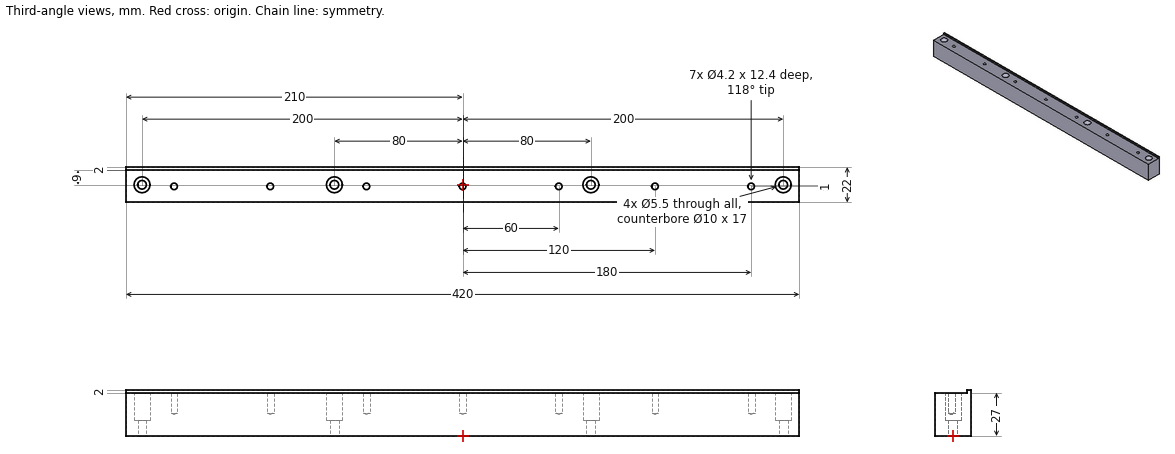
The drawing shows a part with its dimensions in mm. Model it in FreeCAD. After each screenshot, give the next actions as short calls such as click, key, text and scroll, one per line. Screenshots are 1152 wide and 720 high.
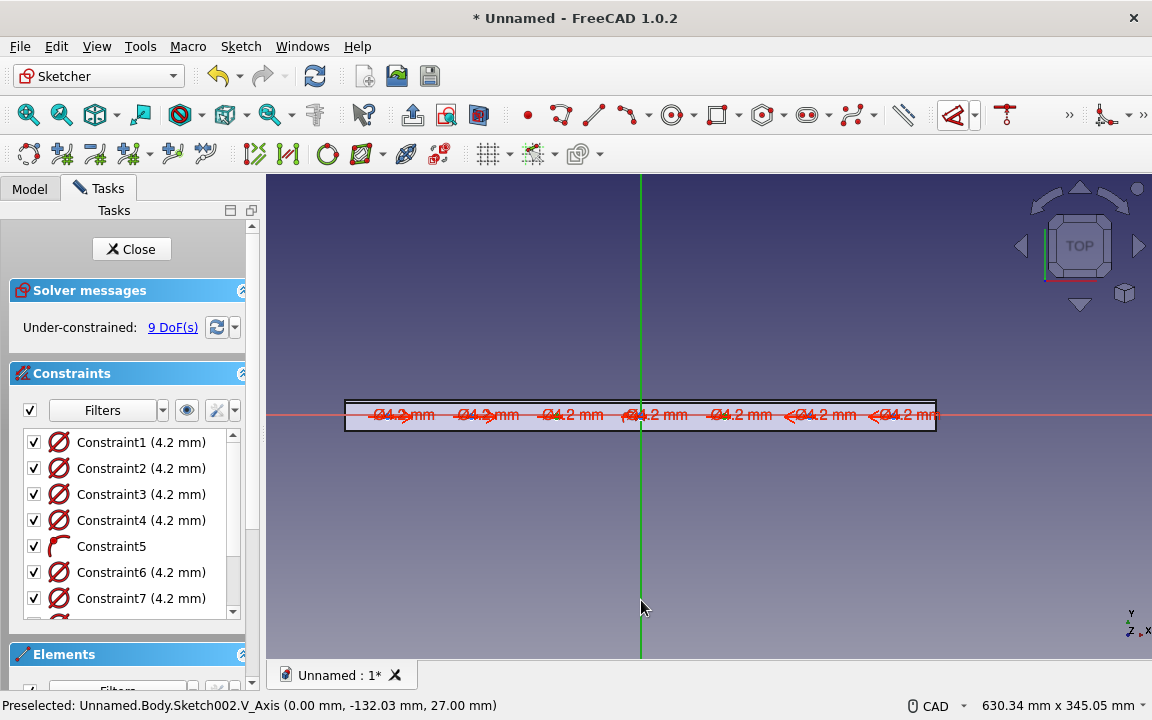
key(s)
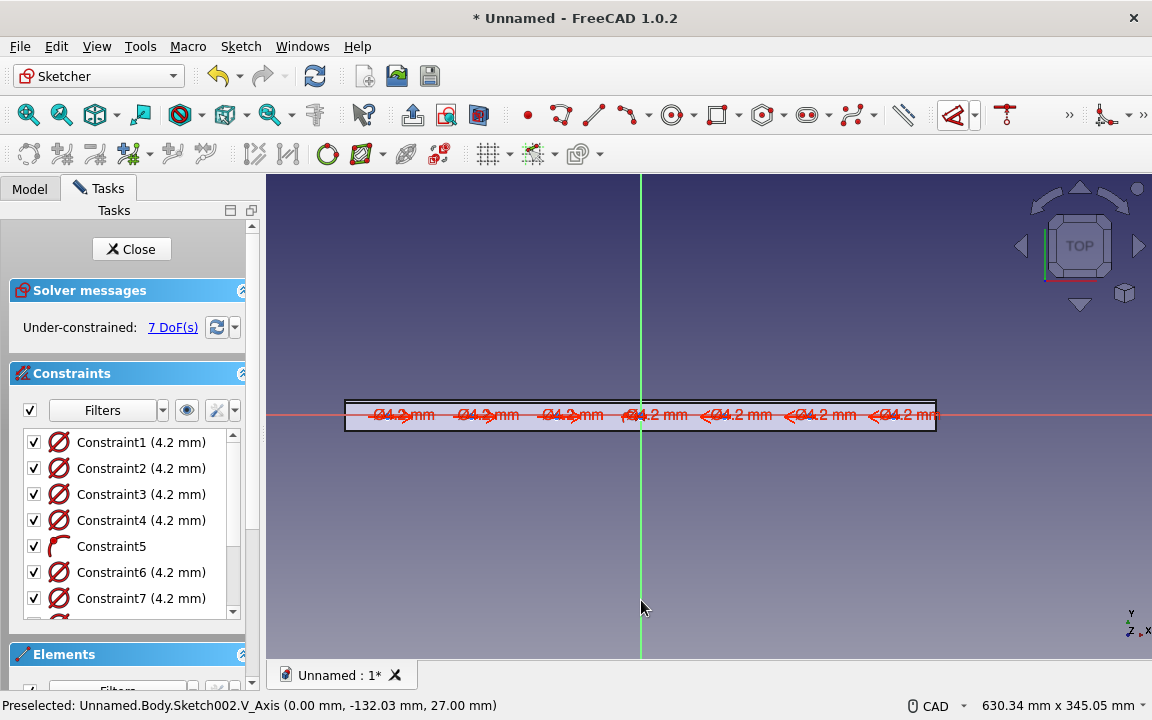
key(d)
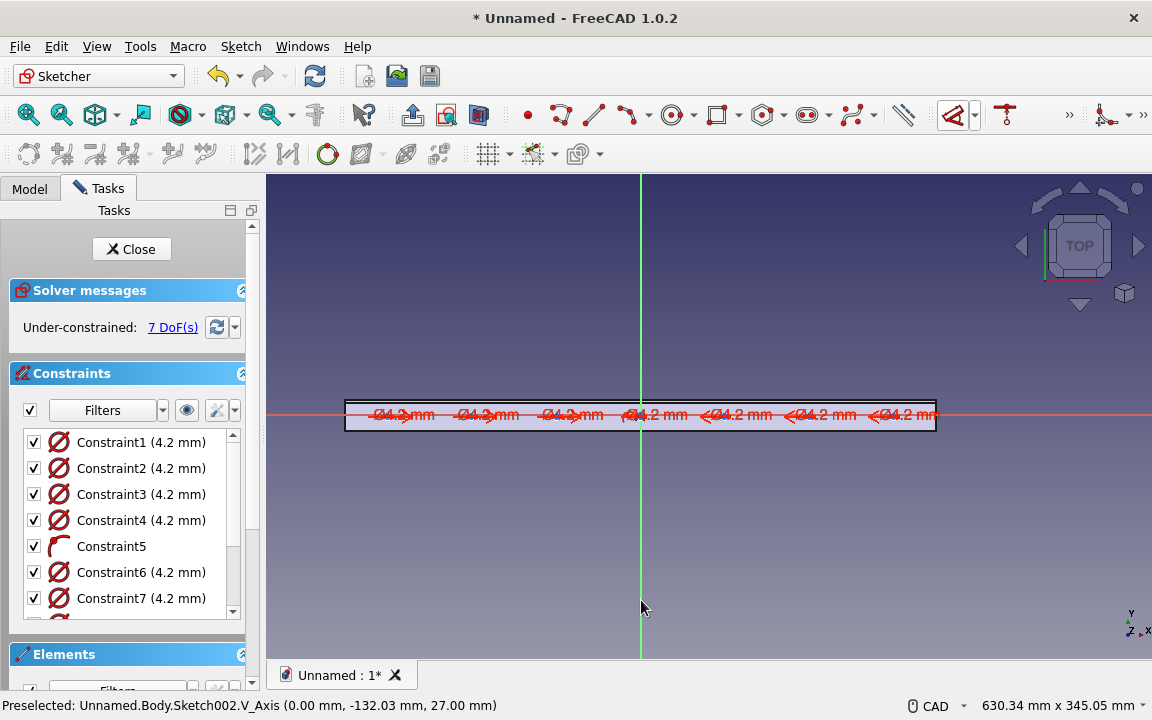
scroll(894, 417, up, 17)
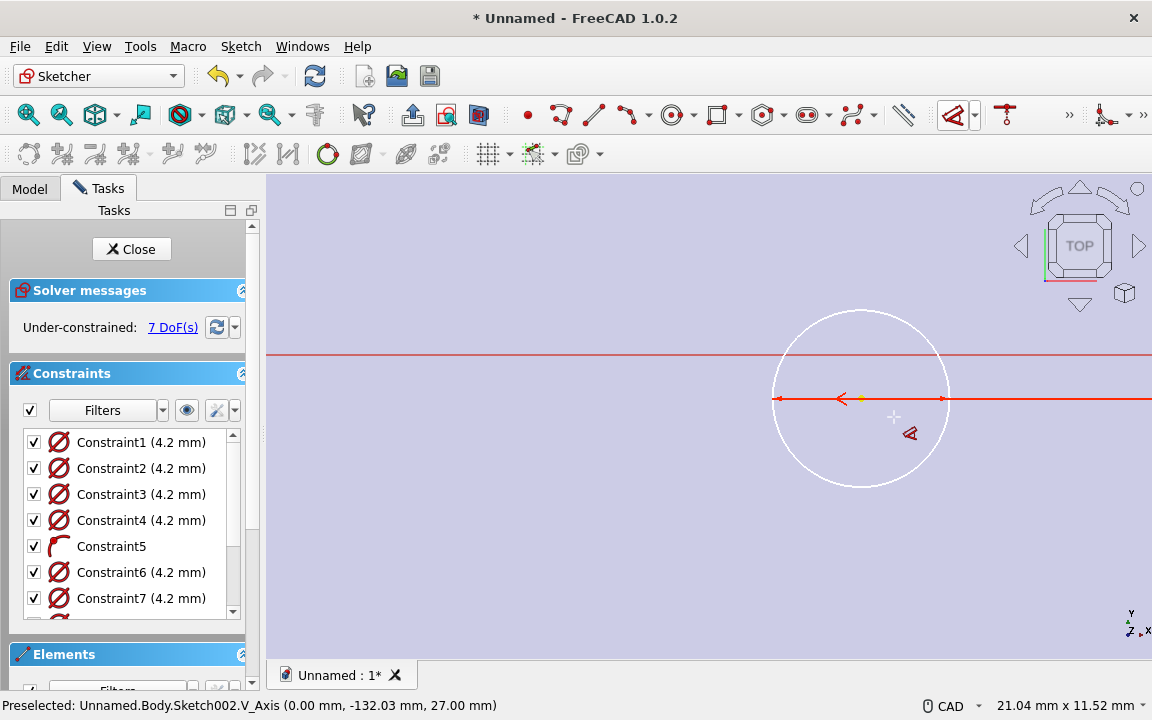
click(861, 399)
click(895, 377)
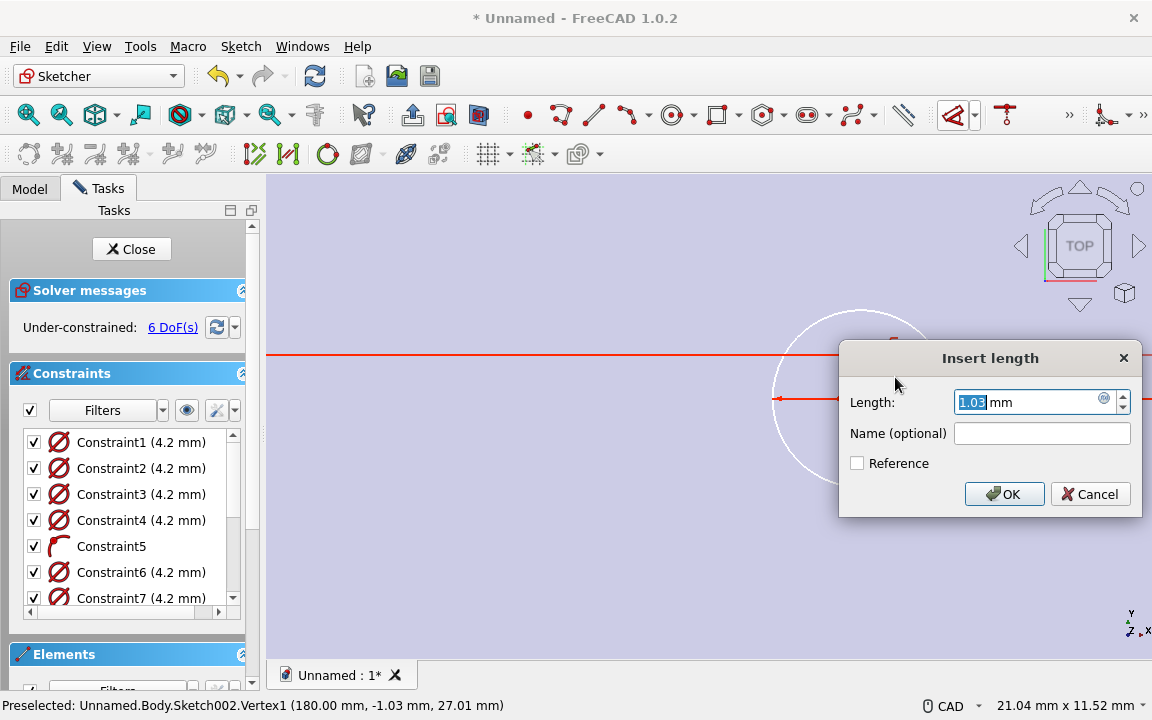
text(1)
key(Return)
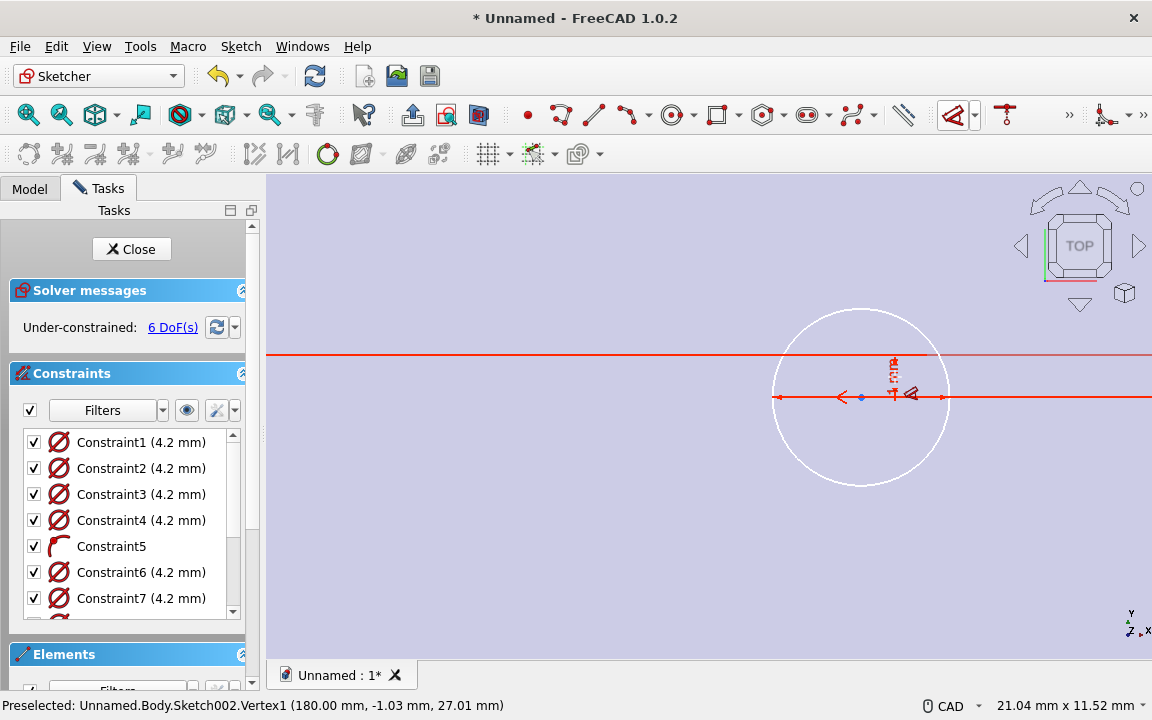
scroll(953, 417, down, 16)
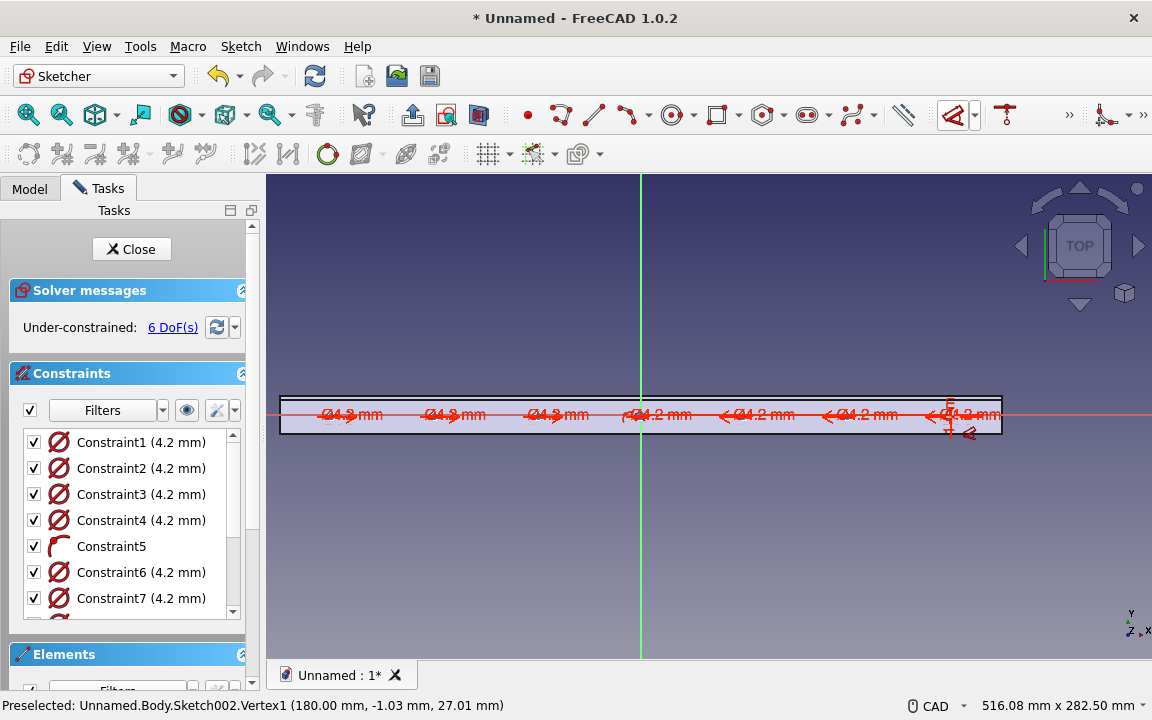
scroll(847, 417, up, 16)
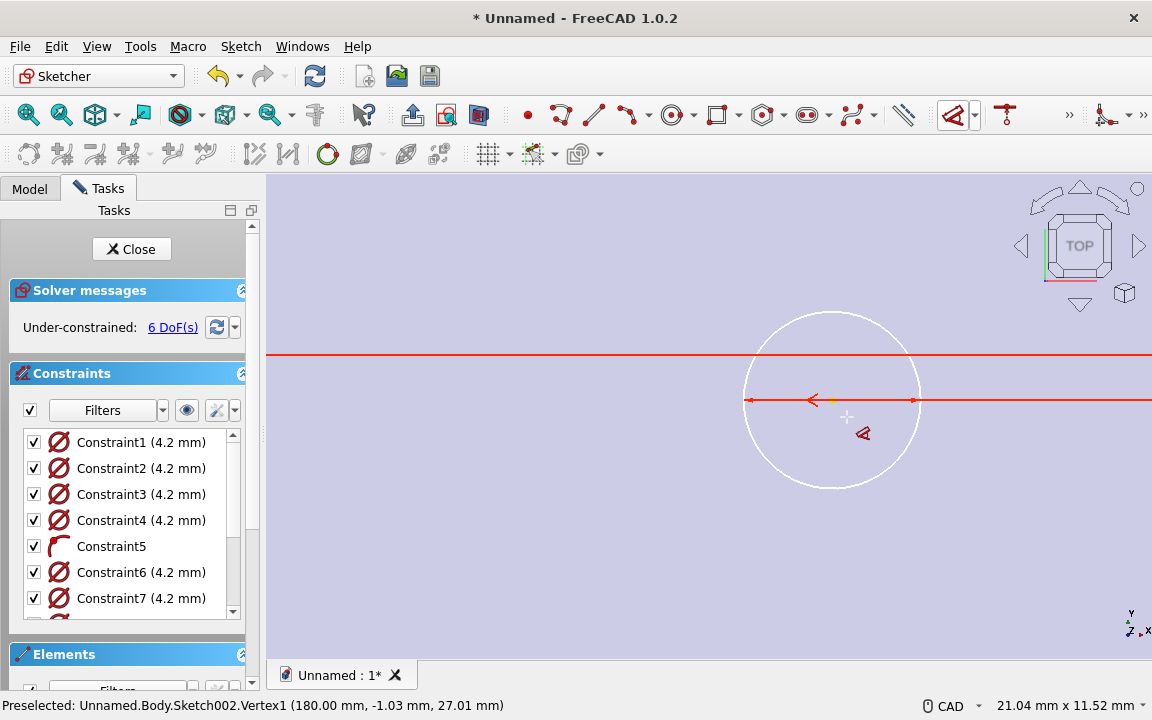
click(832, 400)
click(866, 378)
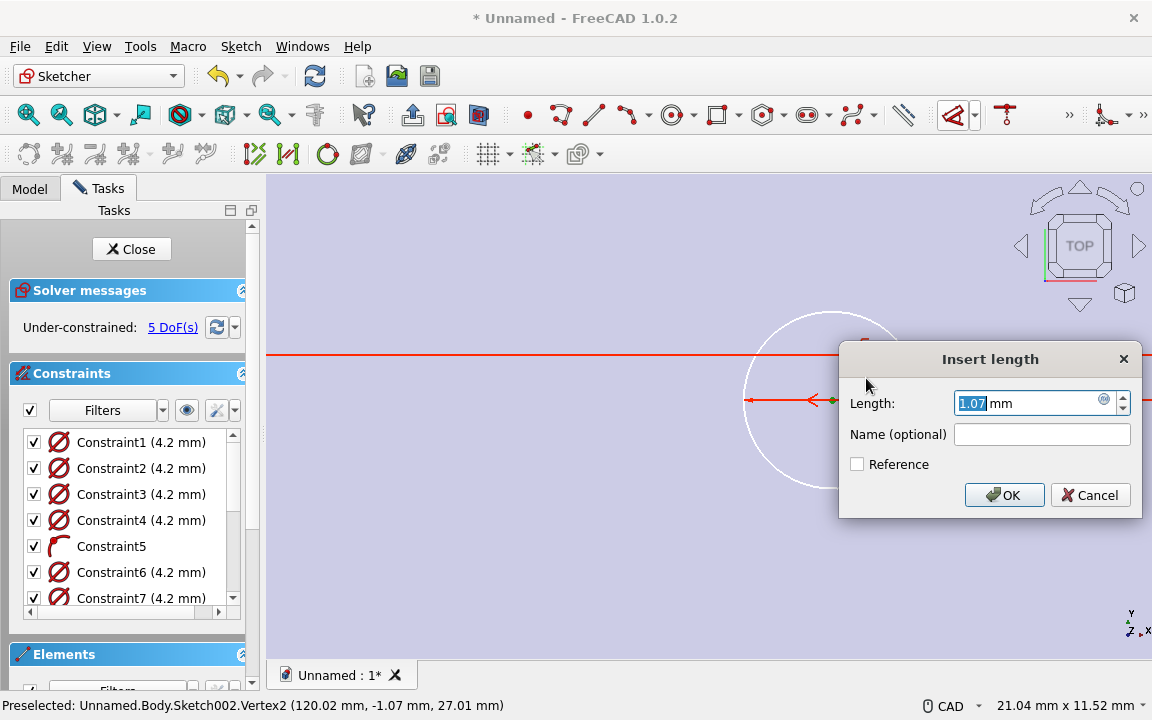
text(1)
key(Return)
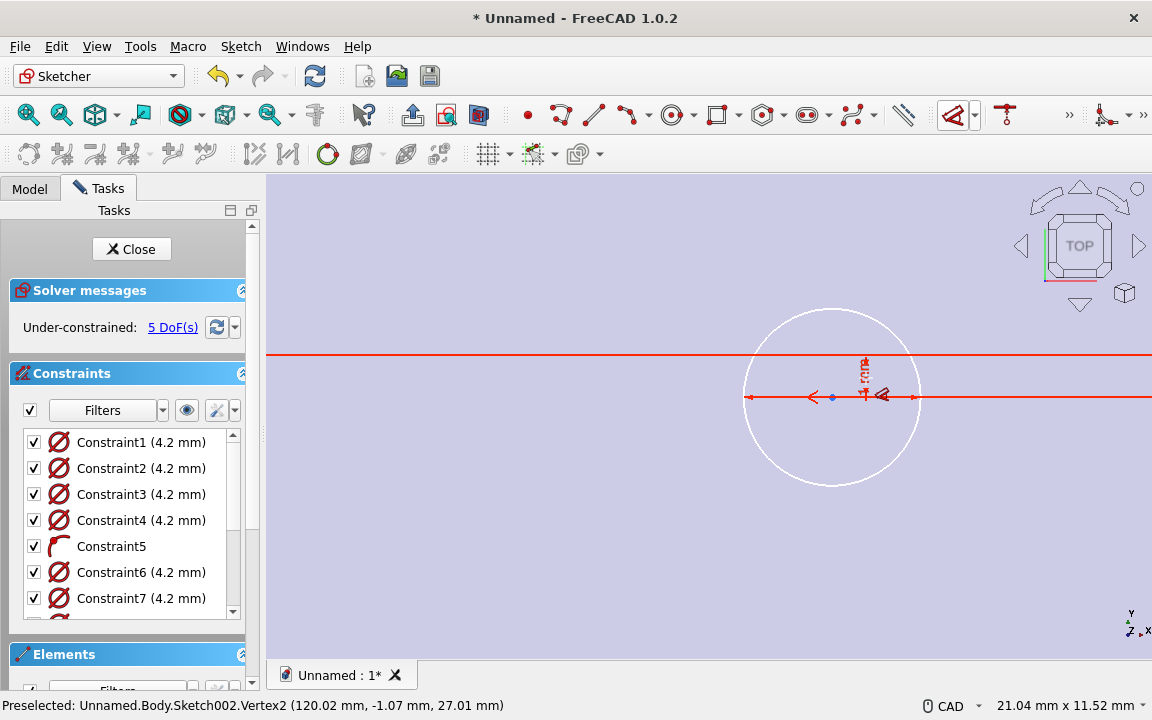
scroll(847, 417, down, 16)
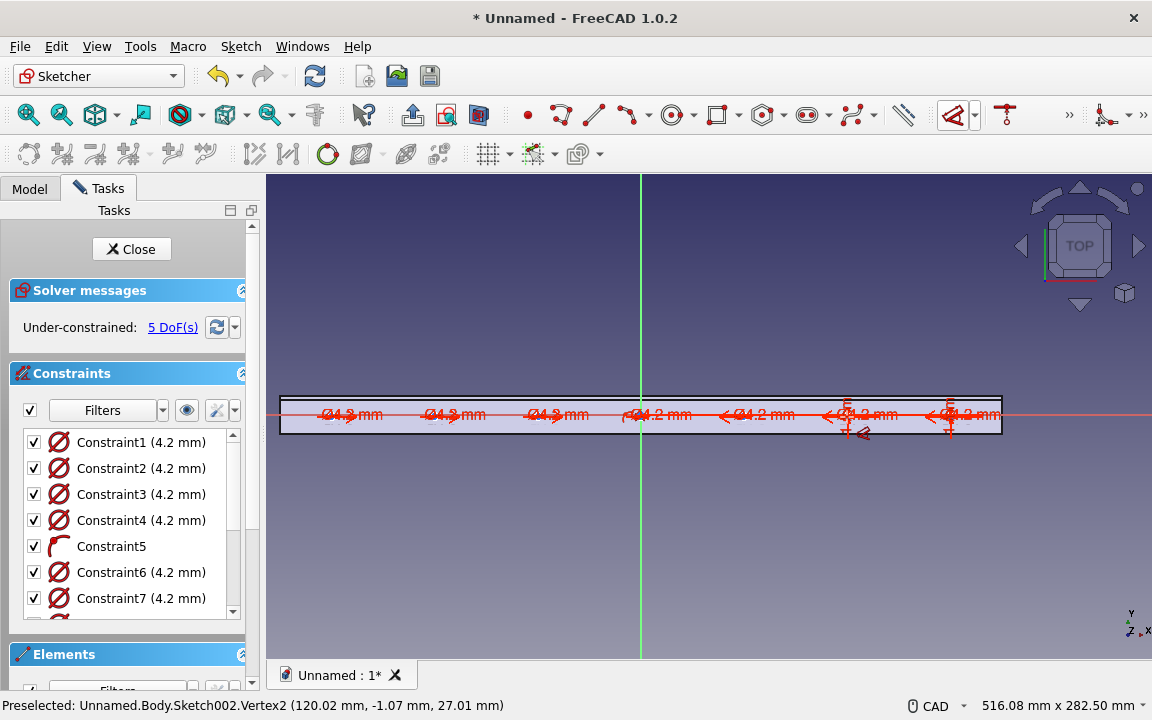
scroll(744, 417, up, 16)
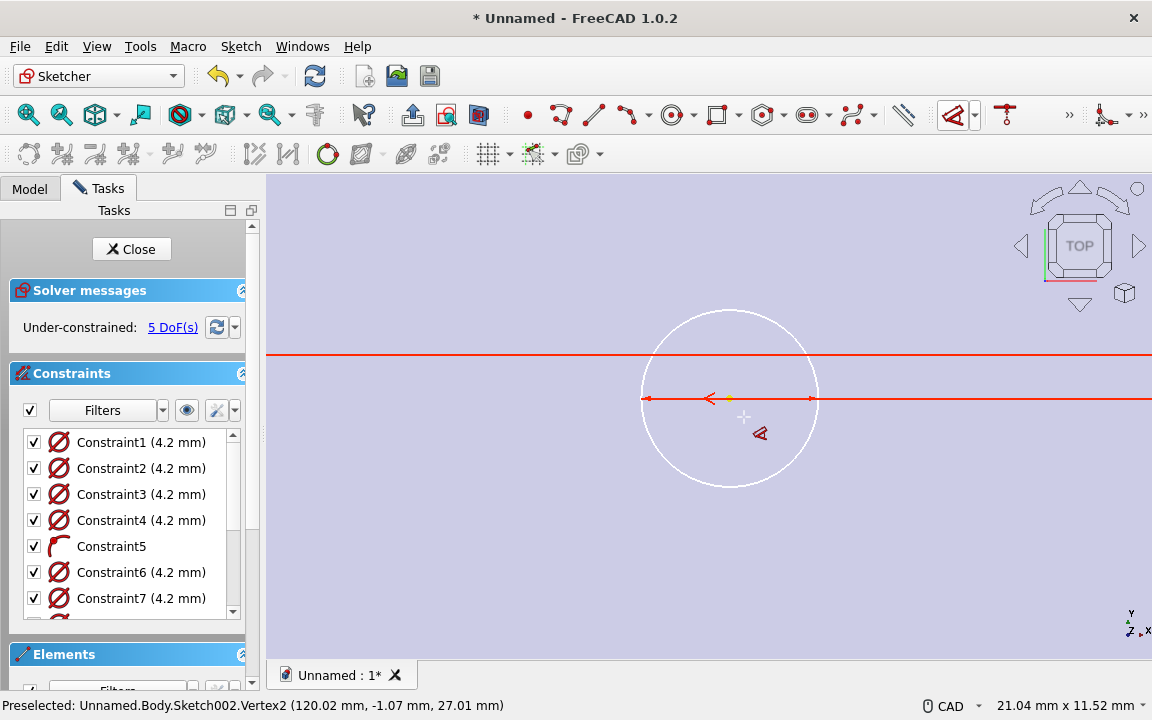
click(730, 399)
click(764, 377)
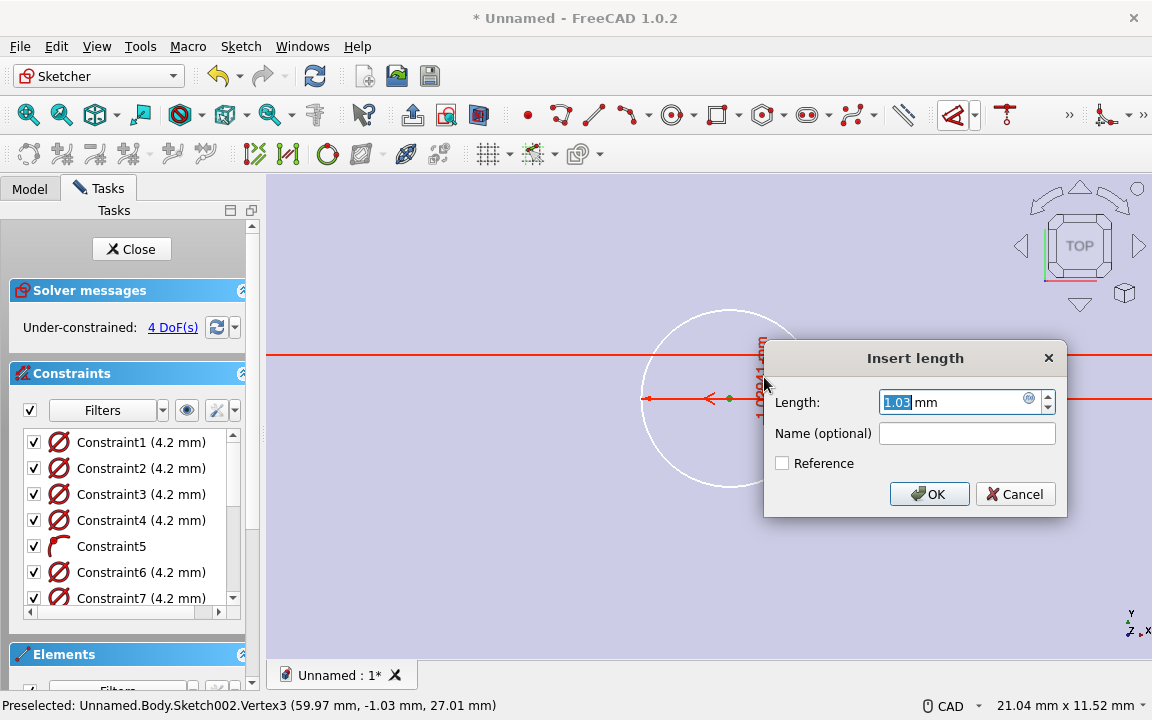
text(1)
key(Return)